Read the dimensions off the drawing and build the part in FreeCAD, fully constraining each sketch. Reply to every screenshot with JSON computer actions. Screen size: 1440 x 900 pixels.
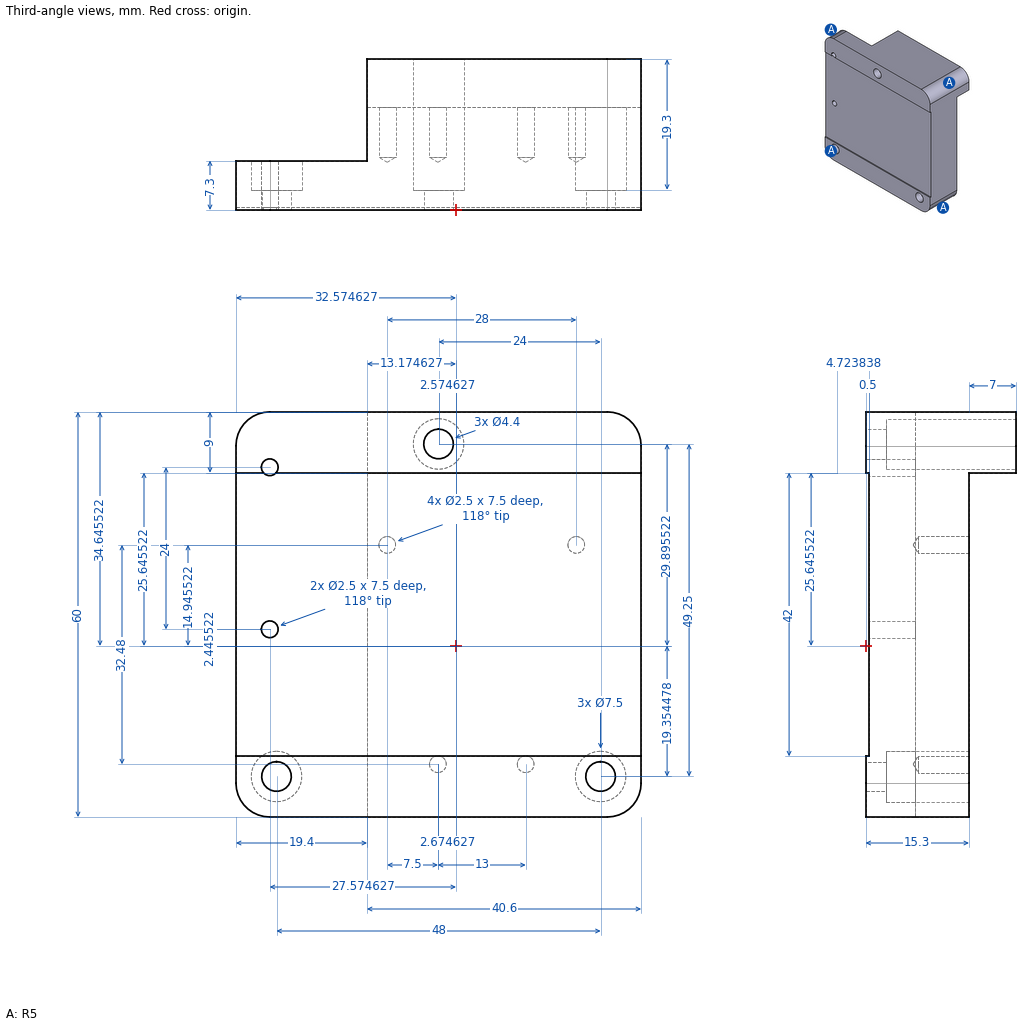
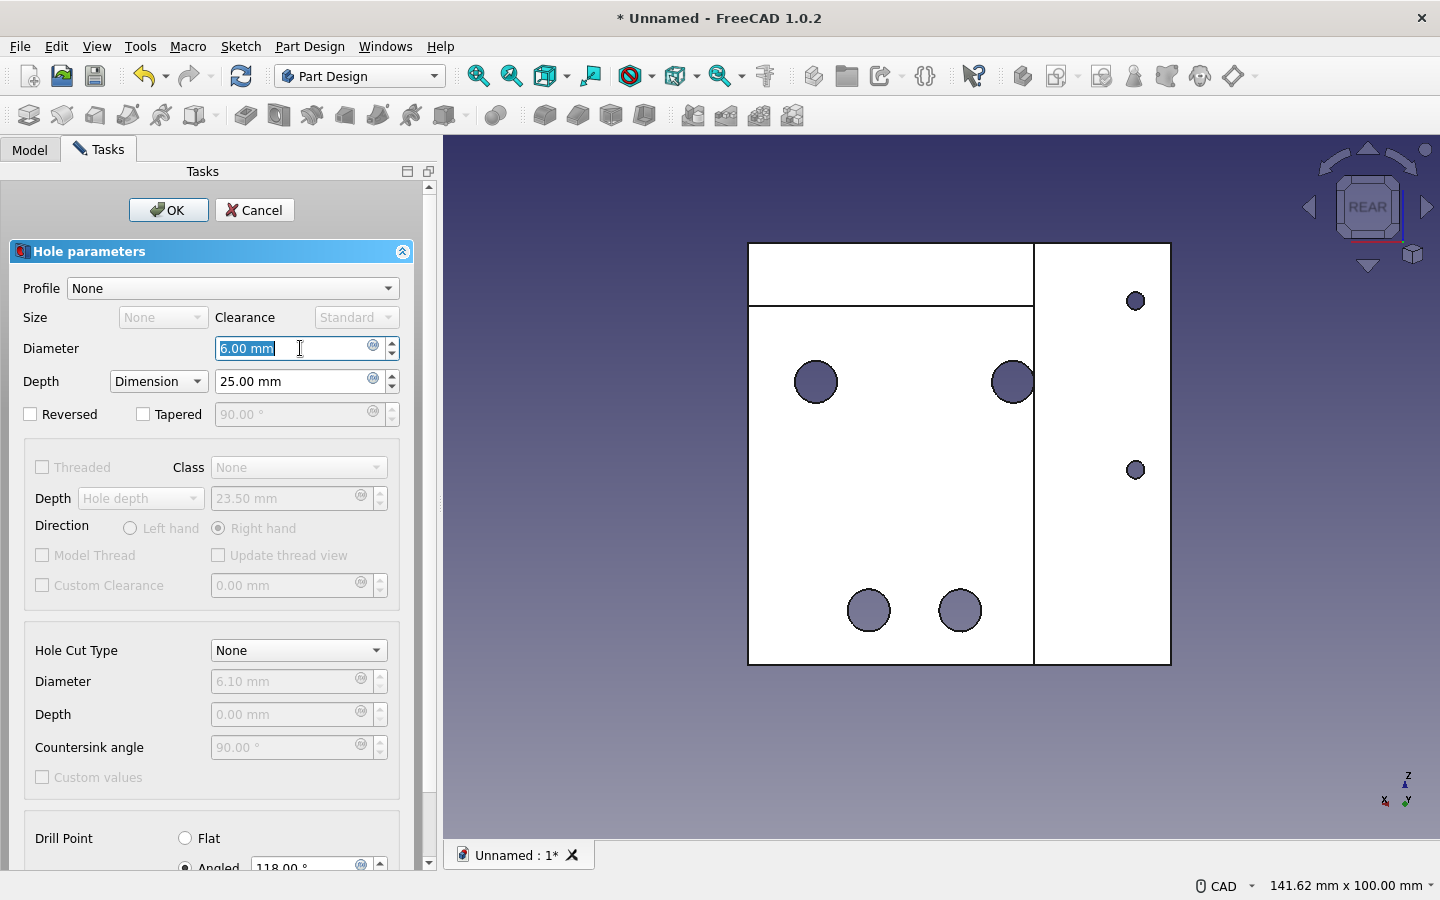
{"action": "type", "text": "2.5"}
{"action": "key", "text": "Tab"}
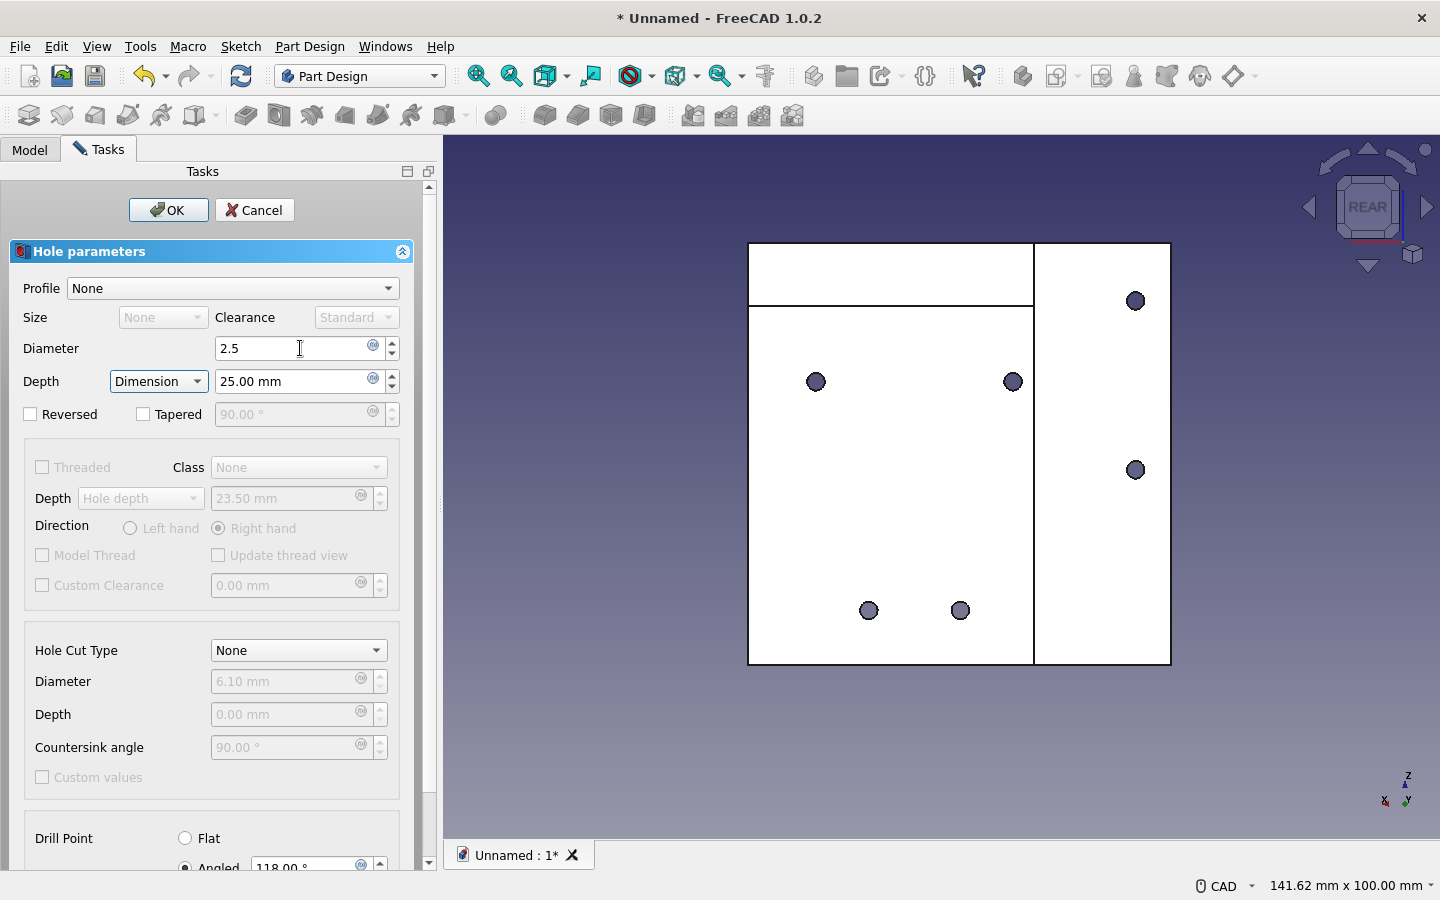
{"action": "triple_click", "coordinate": [300, 382]}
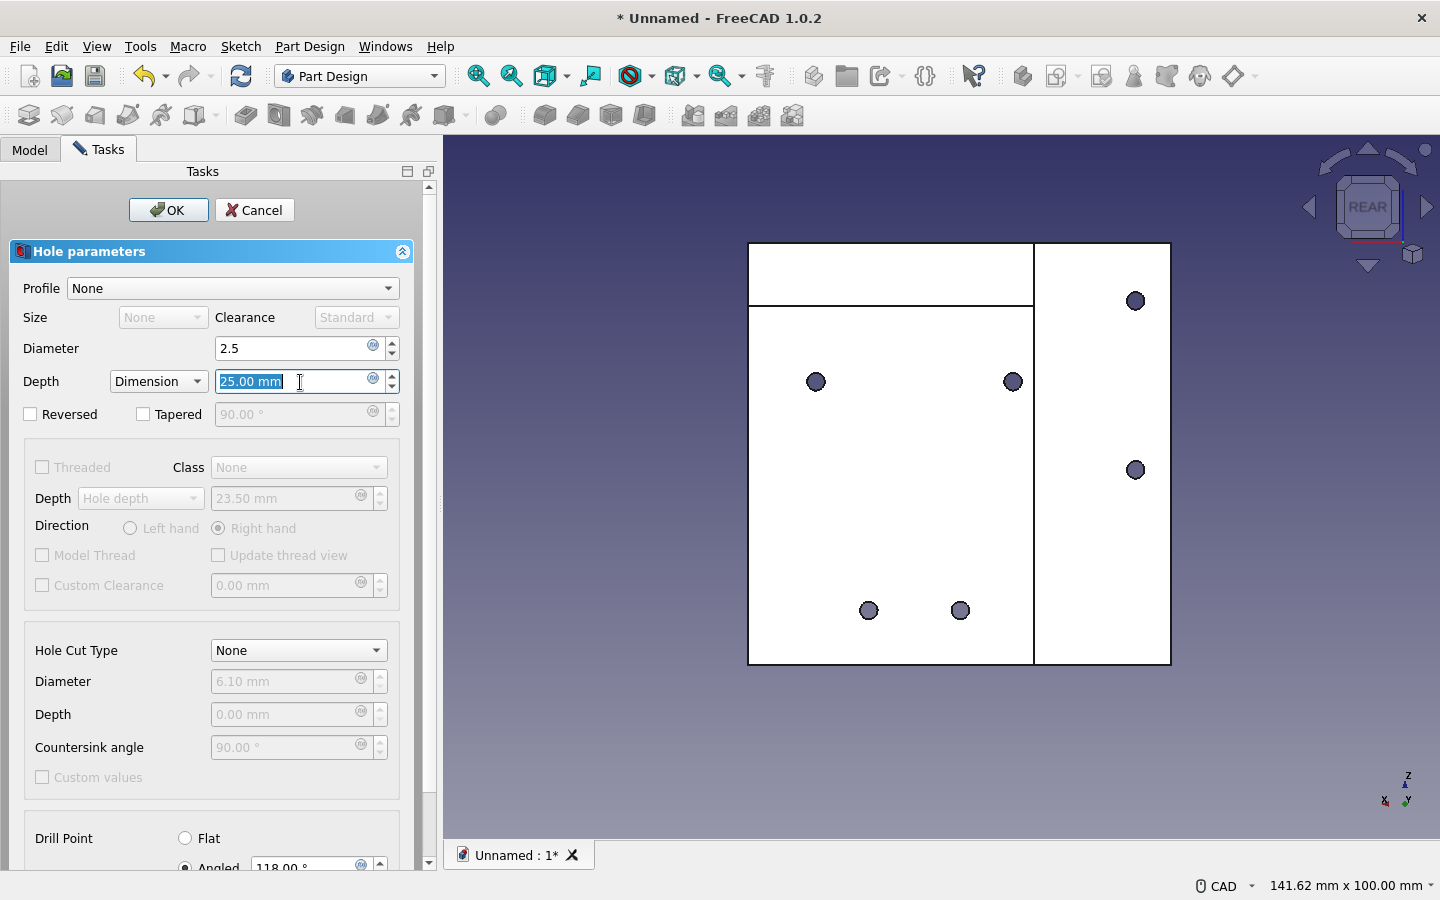
{"action": "type", "text": "7.5"}
{"action": "key", "text": "Tab"}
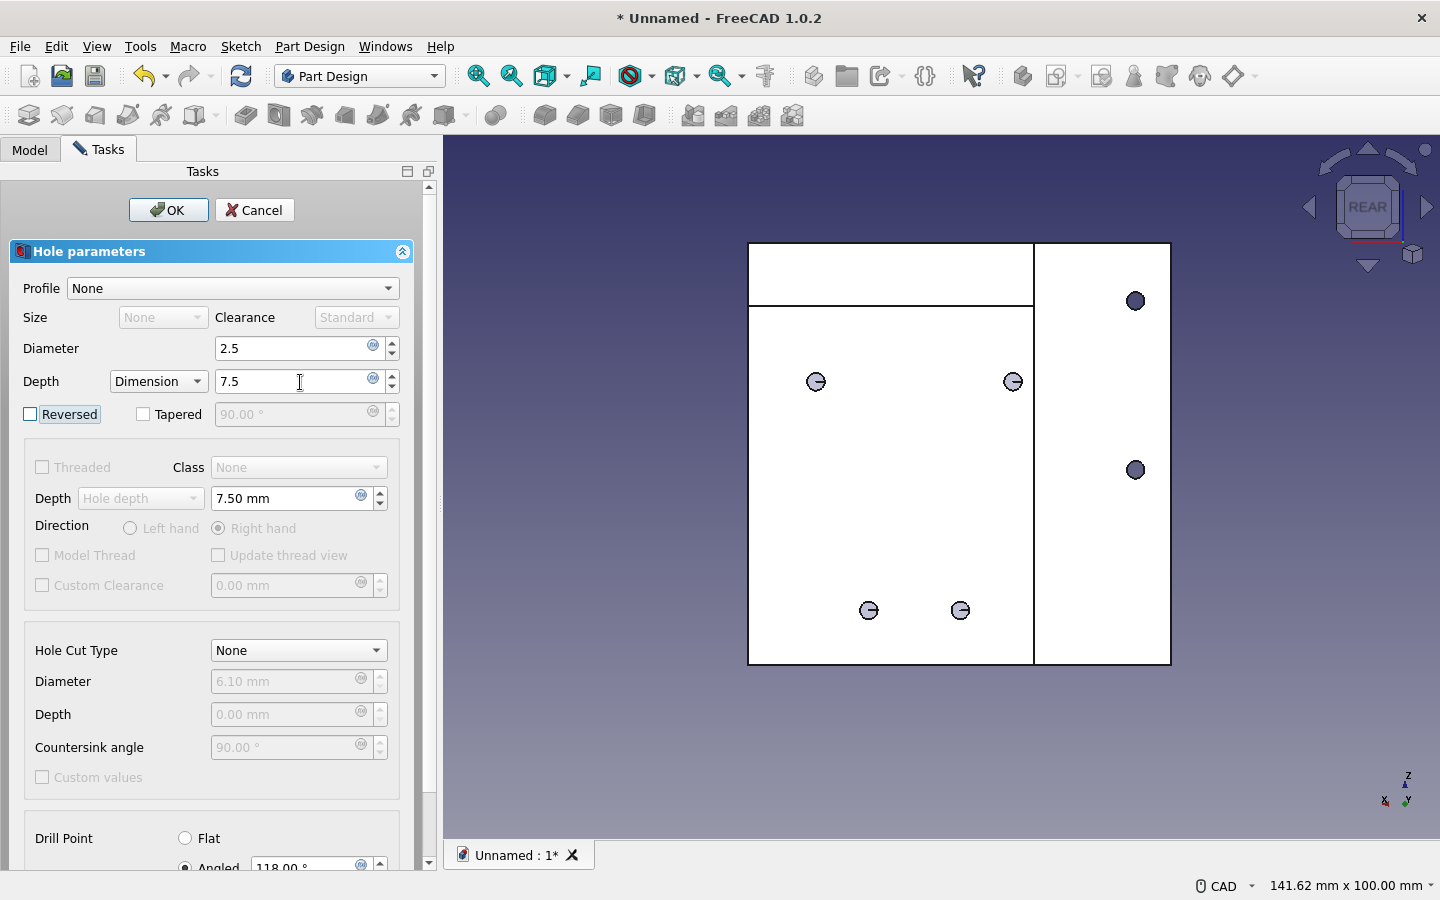
{"action": "left_click", "coordinate": [169, 210]}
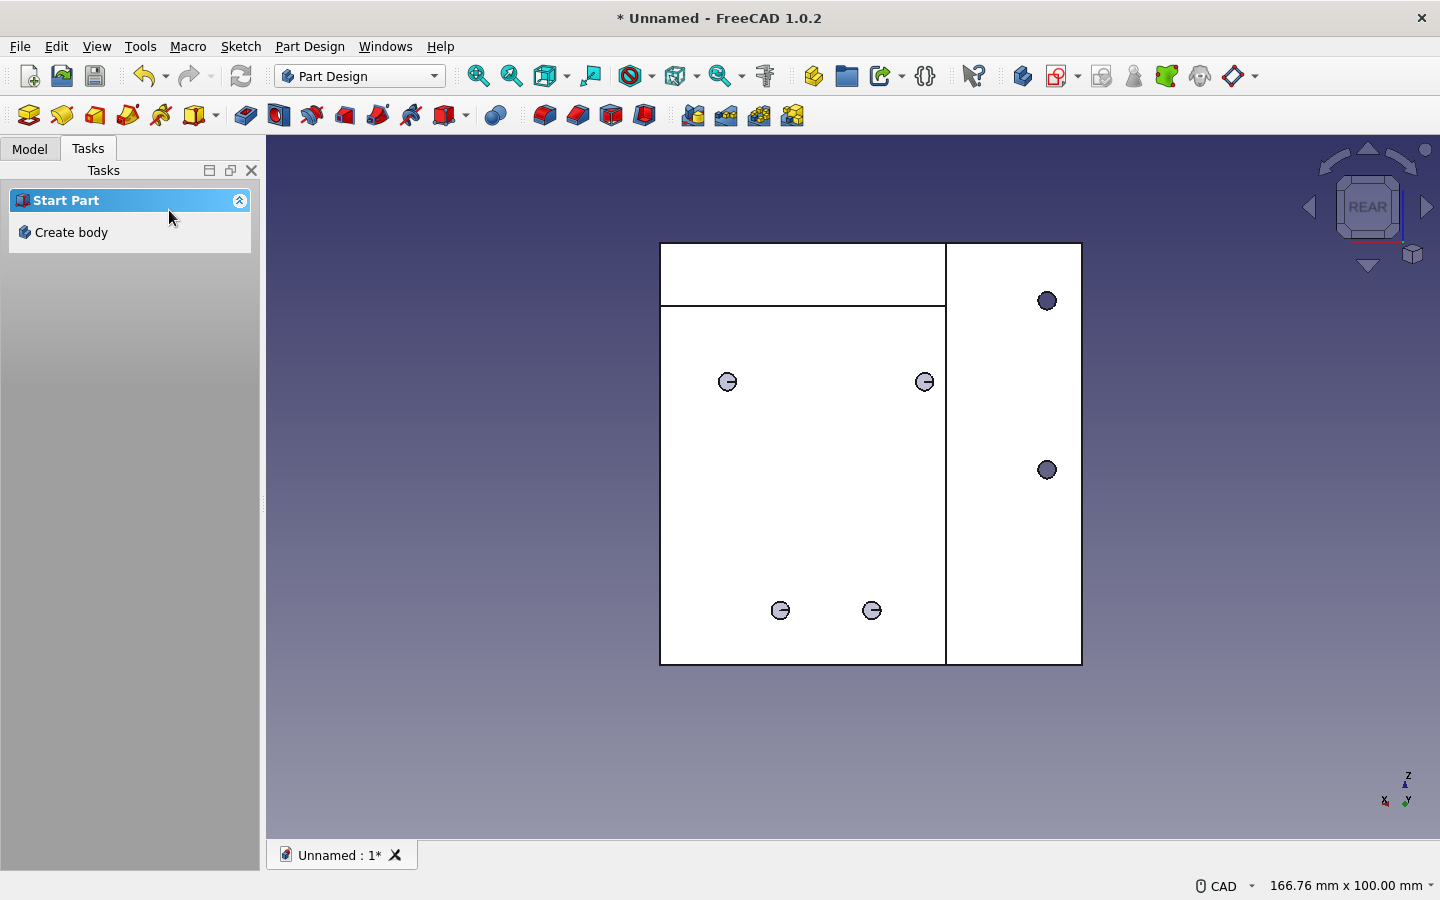
{"action": "key", "text": "0"}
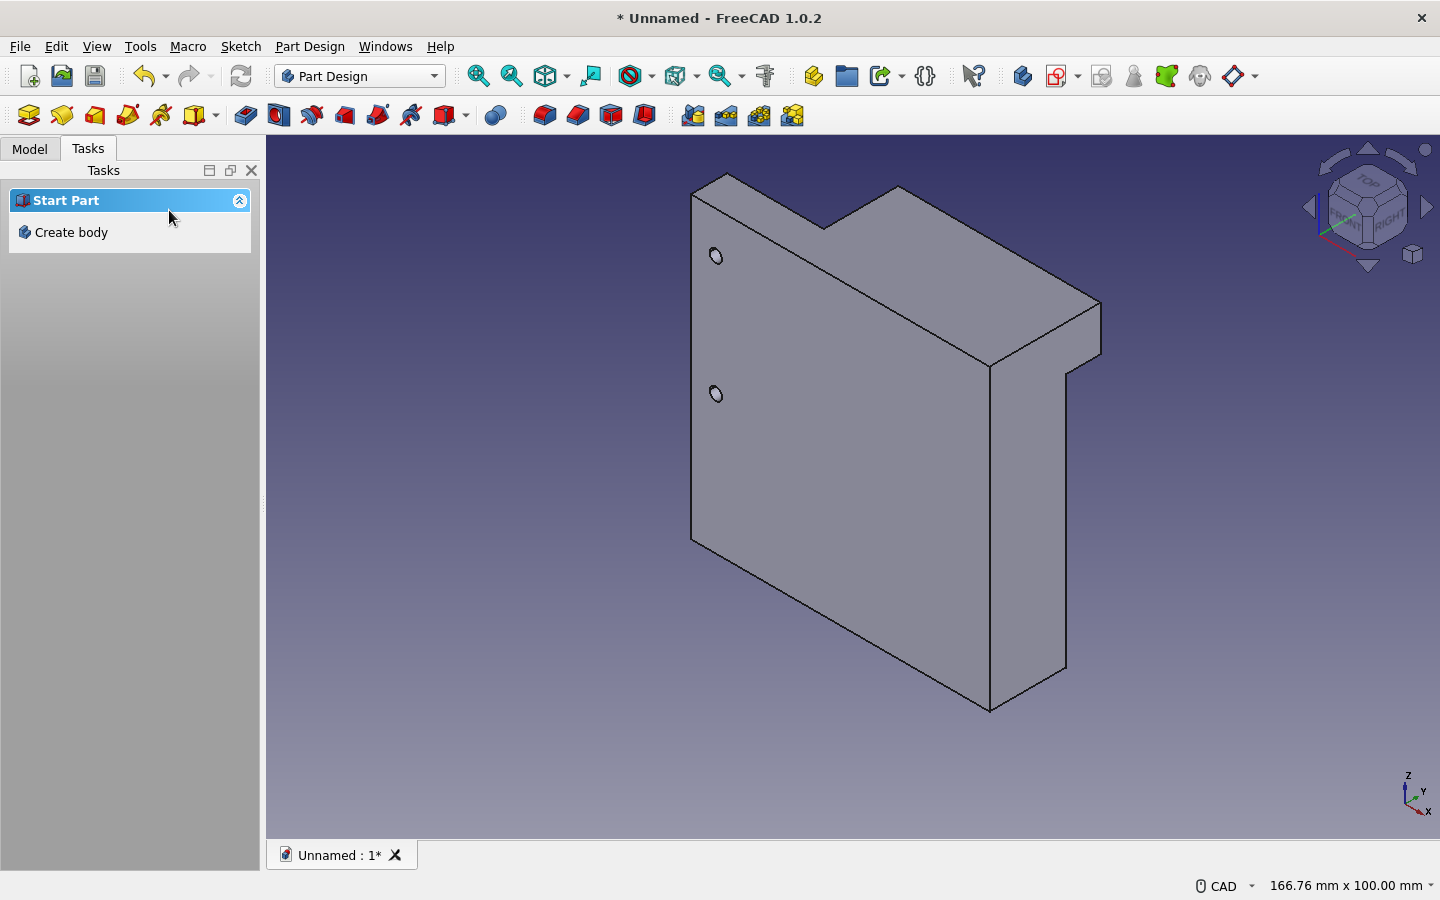
{"action": "key", "text": "v f"}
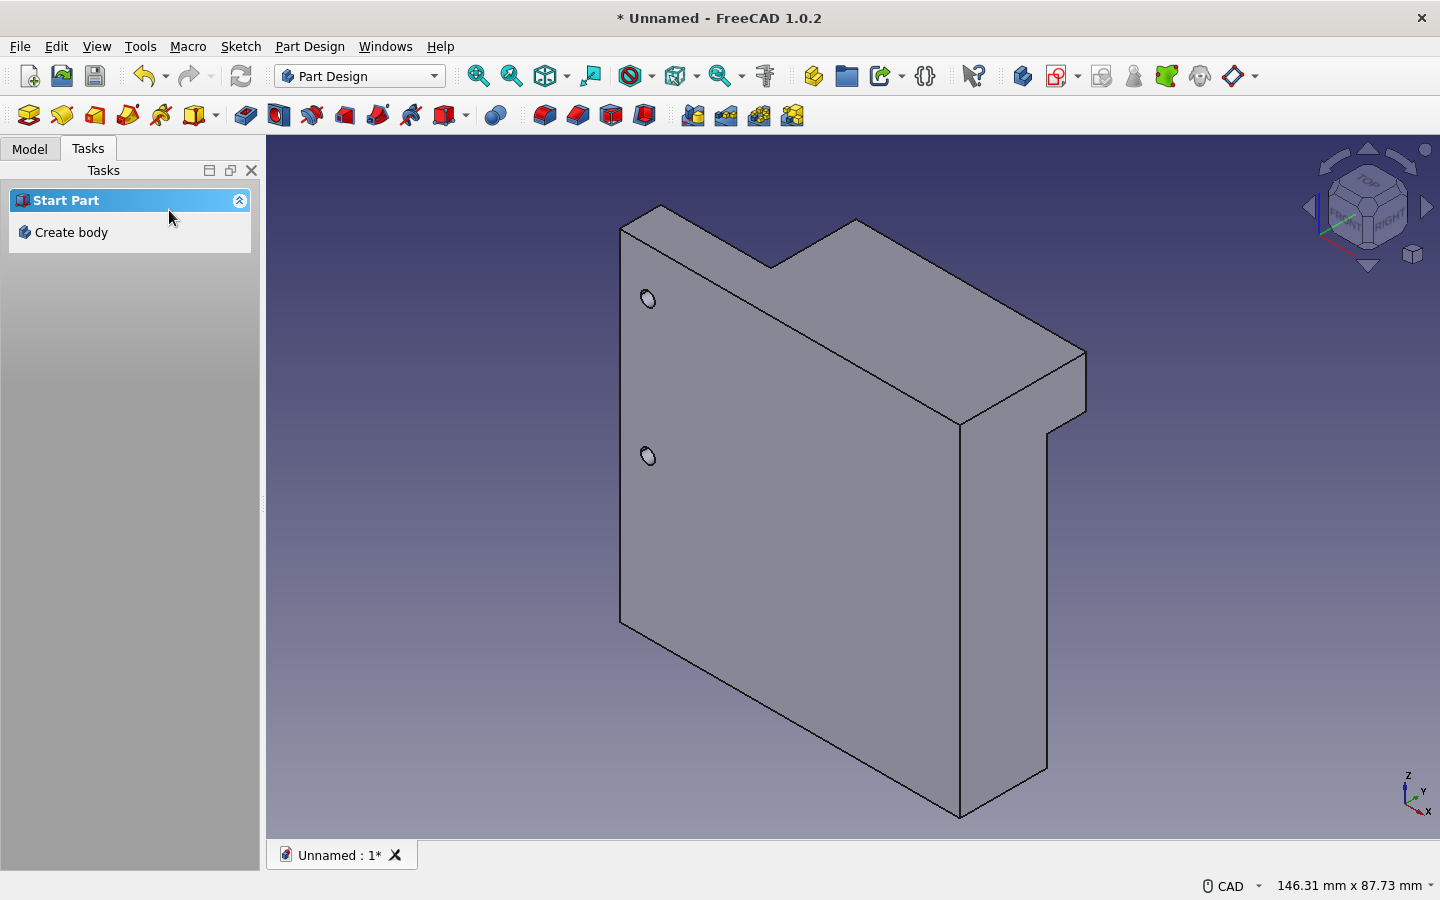
{"action": "left_click", "coordinate": [1023, 388]}